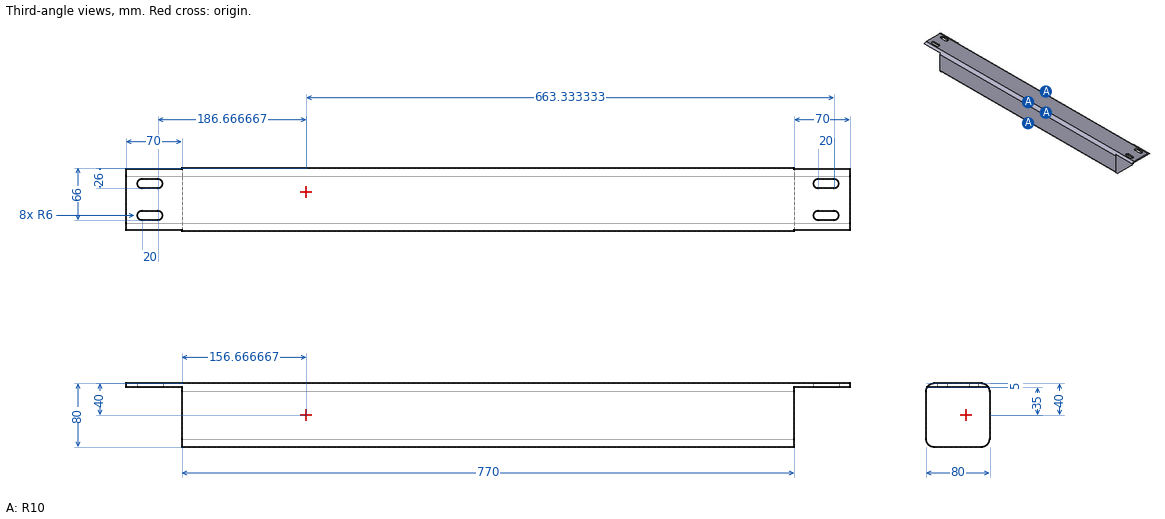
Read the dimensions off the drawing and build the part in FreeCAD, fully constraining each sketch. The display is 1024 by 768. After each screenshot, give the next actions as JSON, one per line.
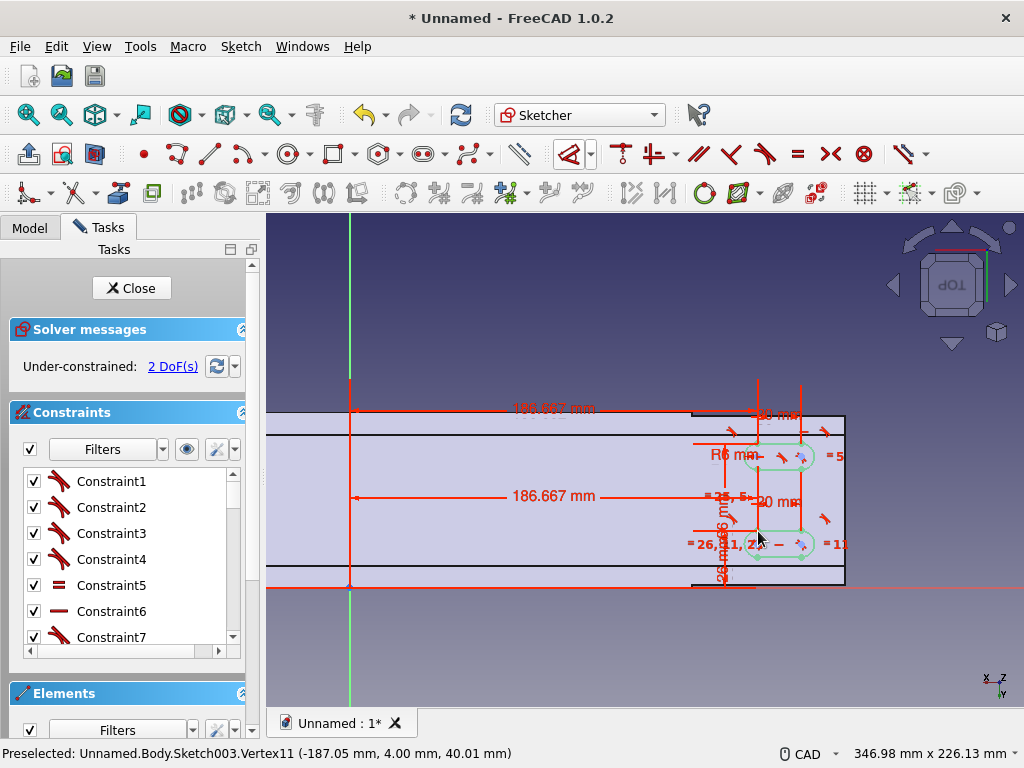
{"action": "scroll", "coordinate": [760, 446], "scroll_direction": "down", "scroll_amount": 8}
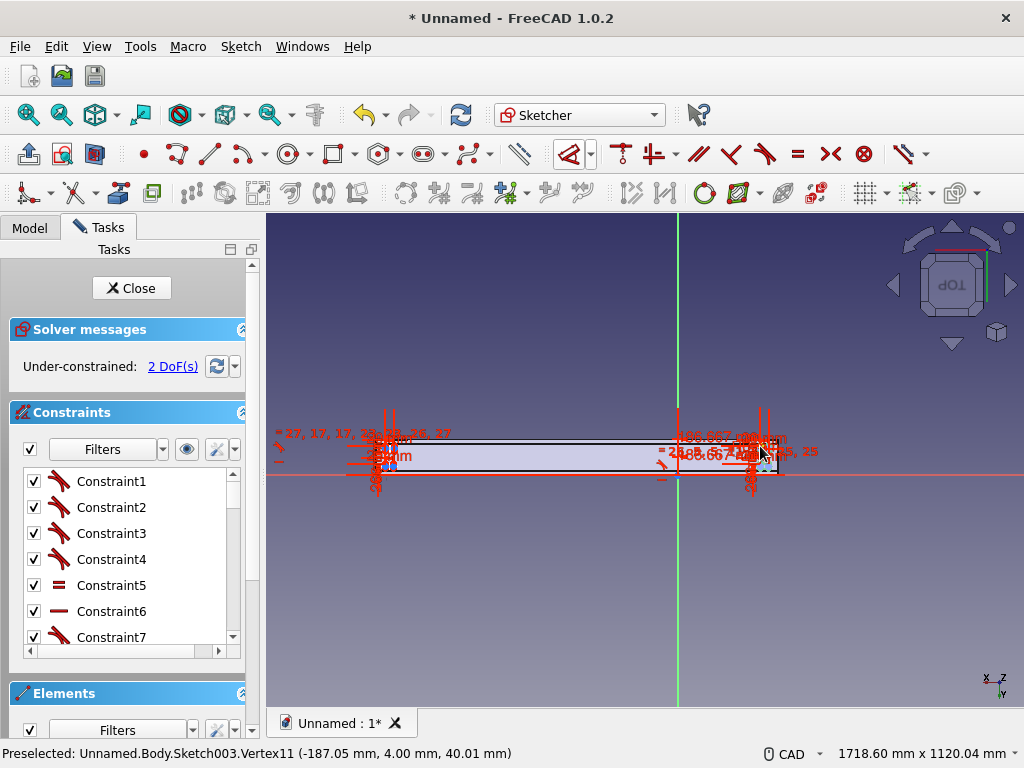
{"action": "scroll", "coordinate": [385, 464], "scroll_direction": "up", "scroll_amount": 8}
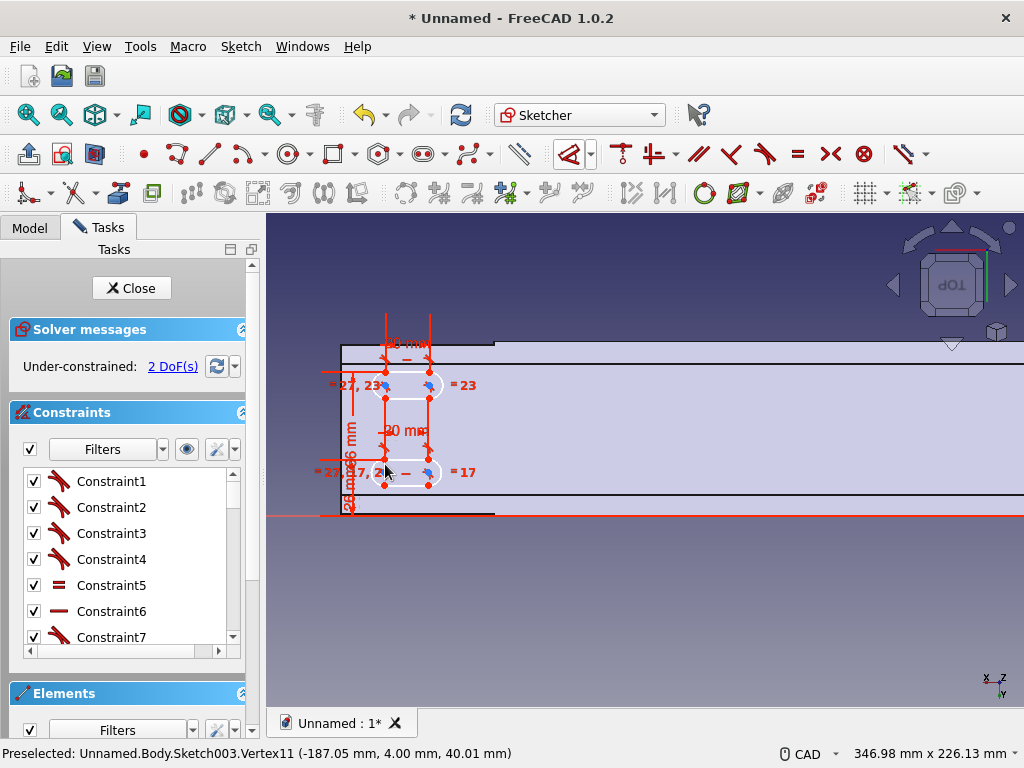
{"action": "left_click", "coordinate": [385, 460]}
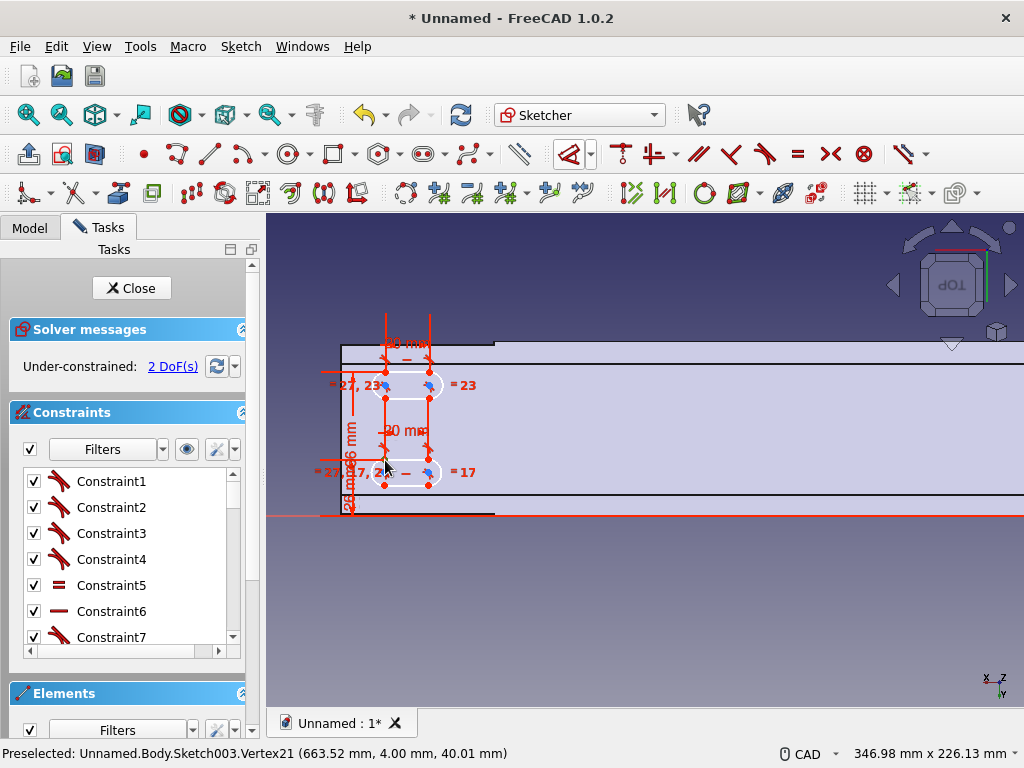
{"action": "left_click", "coordinate": [590, 154]}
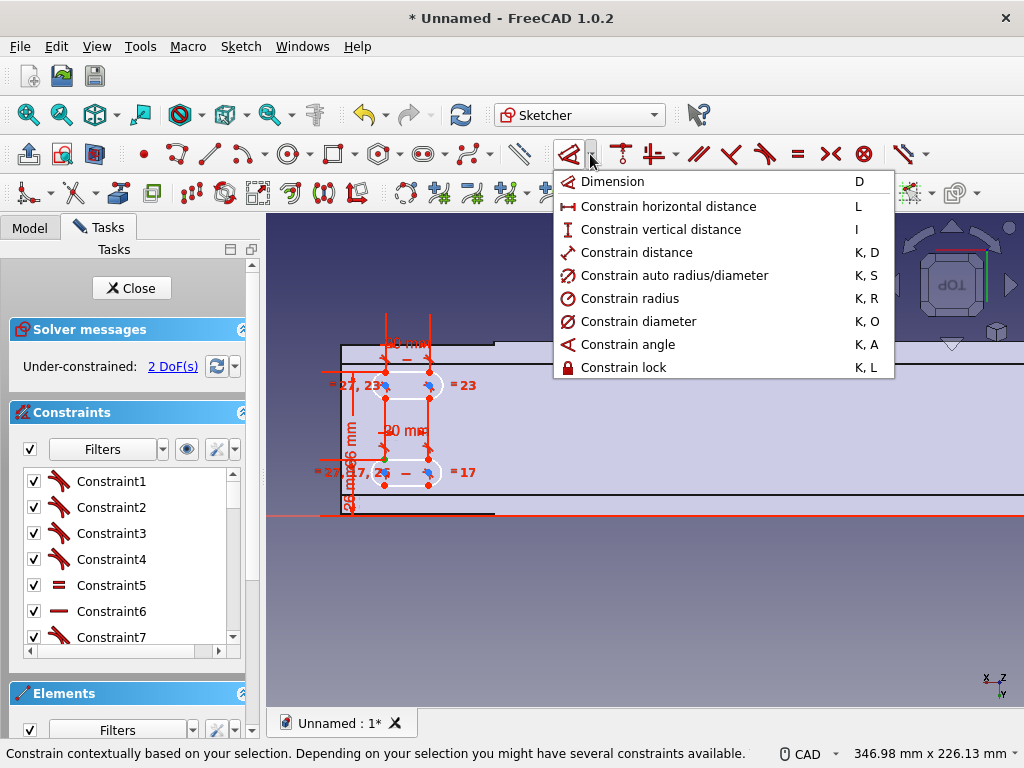
{"action": "left_click", "coordinate": [724, 206]}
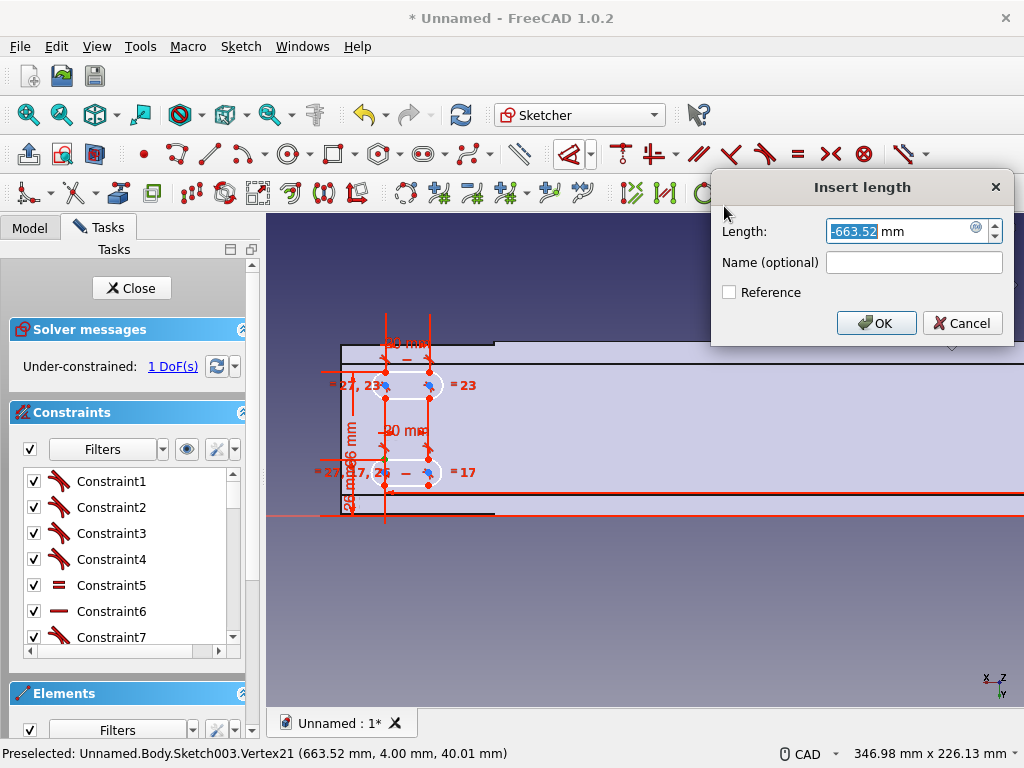
{"action": "type", "text": "-663.333333"}
{"action": "key", "text": "Return"}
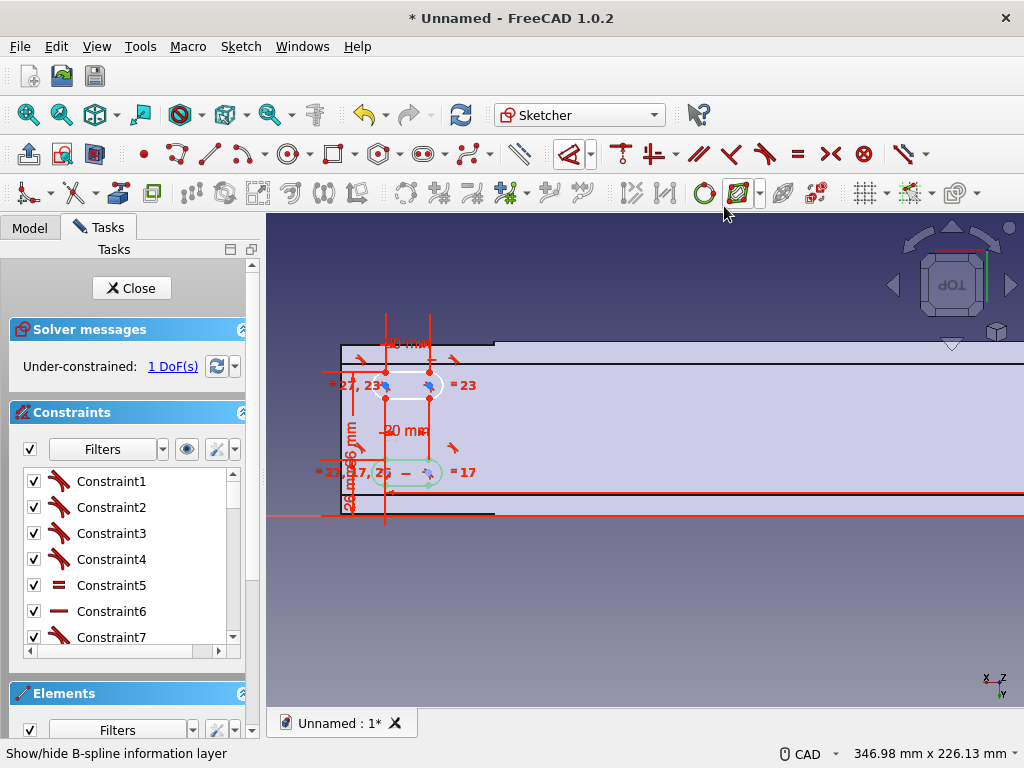
{"action": "left_click", "coordinate": [386, 372]}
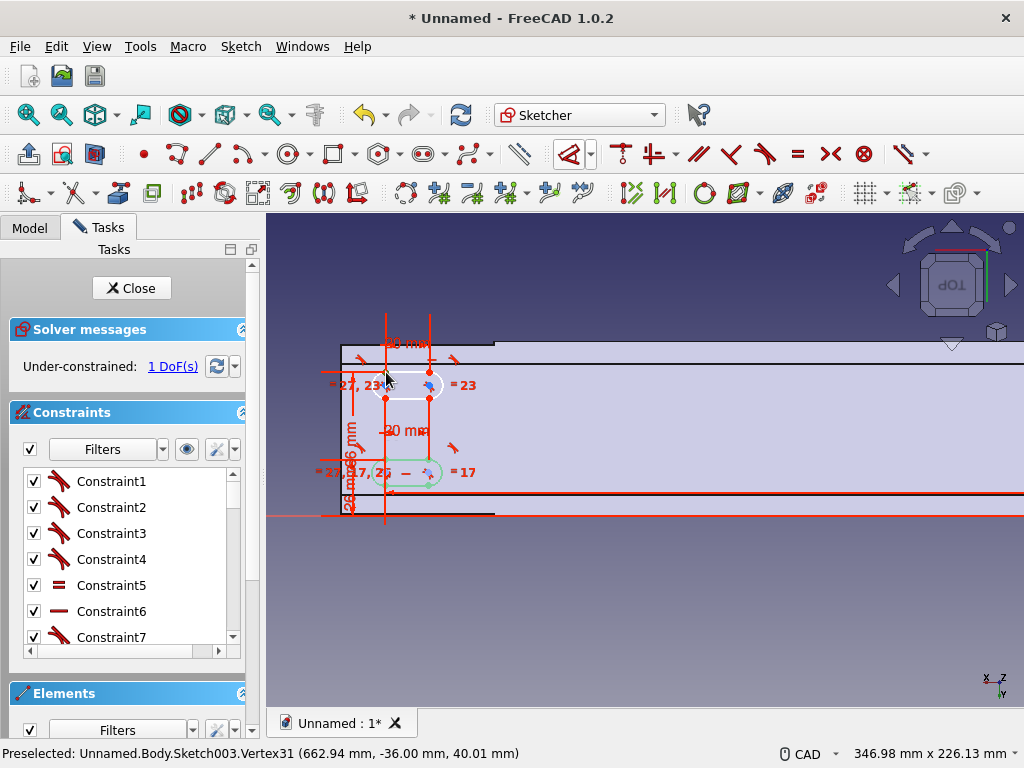
{"action": "left_click", "coordinate": [590, 154]}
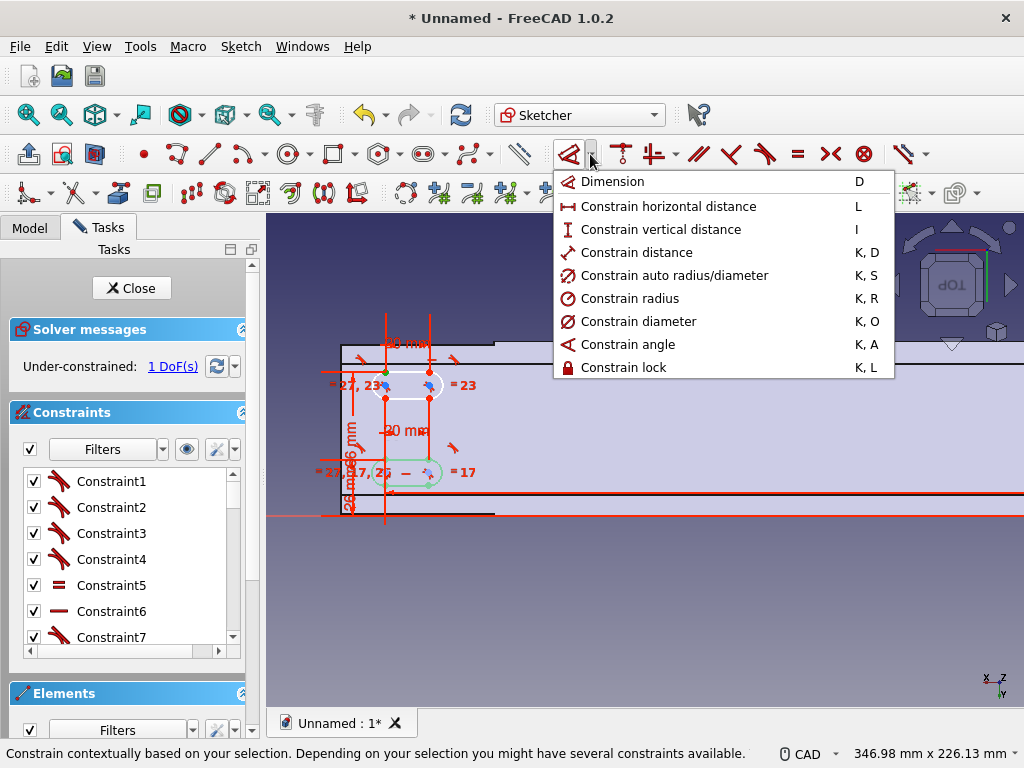
{"action": "left_click", "coordinate": [724, 206]}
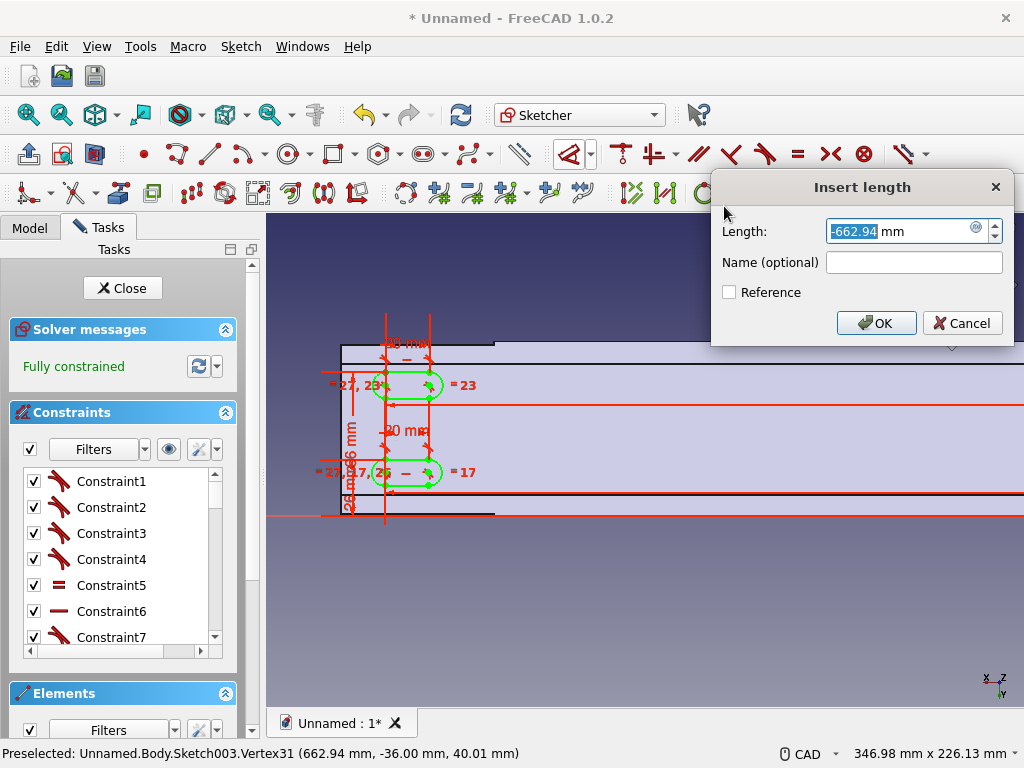
{"action": "type", "text": "-663.333333"}
{"action": "key", "text": "Return"}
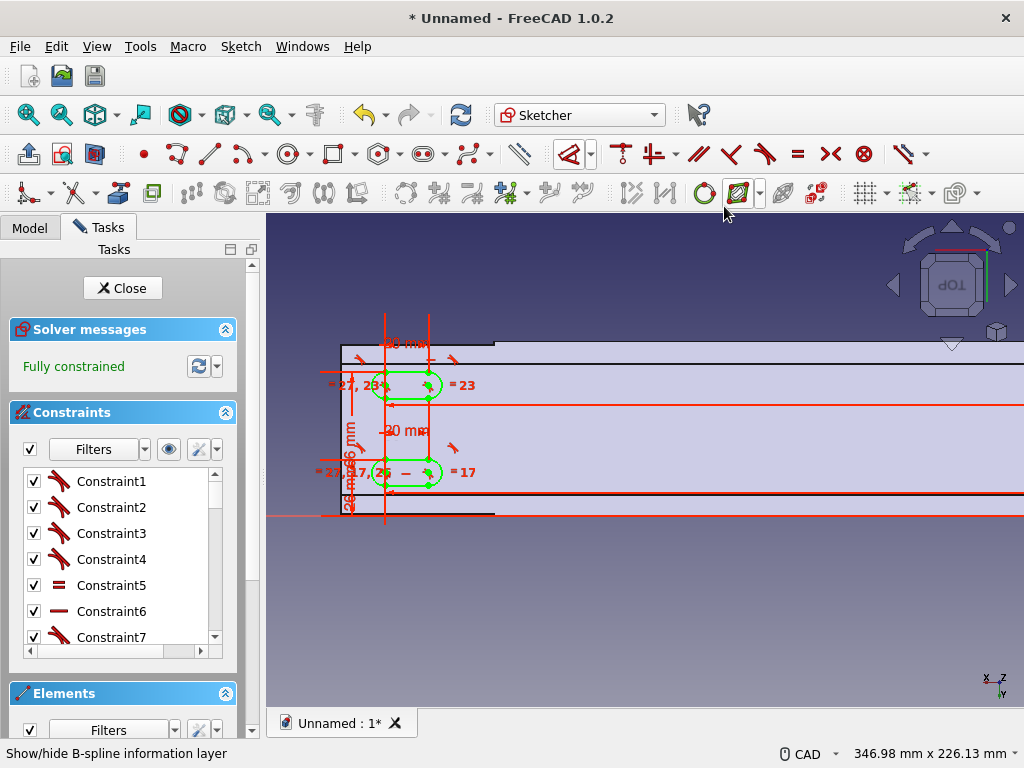
{"action": "left_click", "coordinate": [123, 288]}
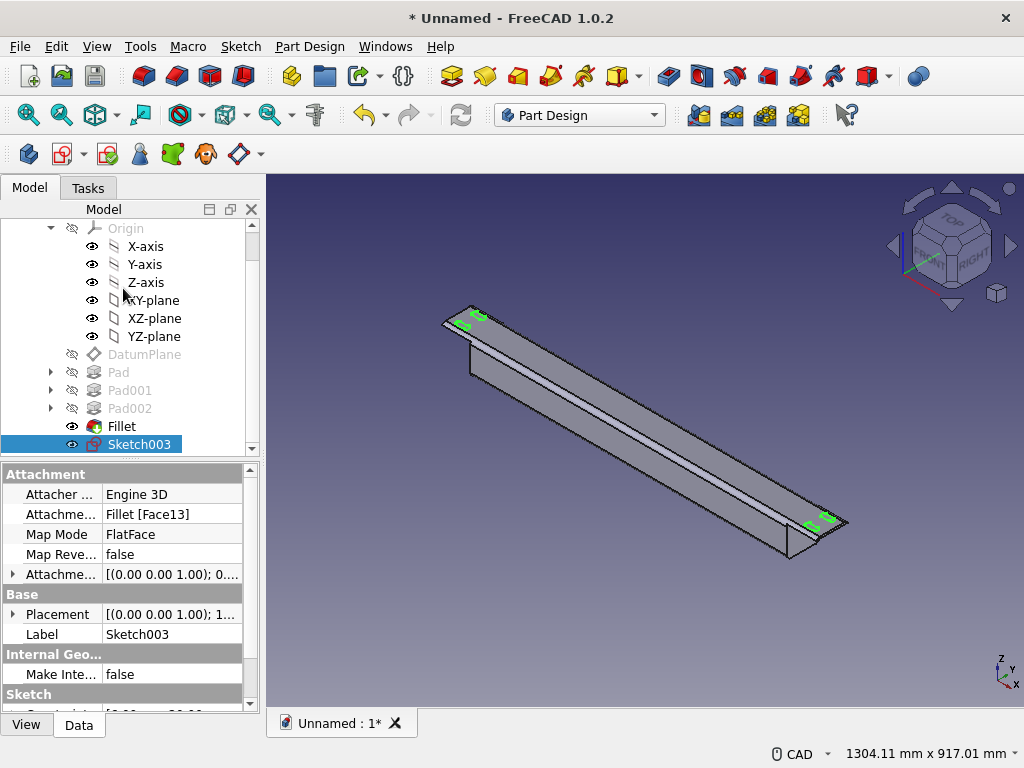
{"action": "left_click", "coordinate": [669, 76]}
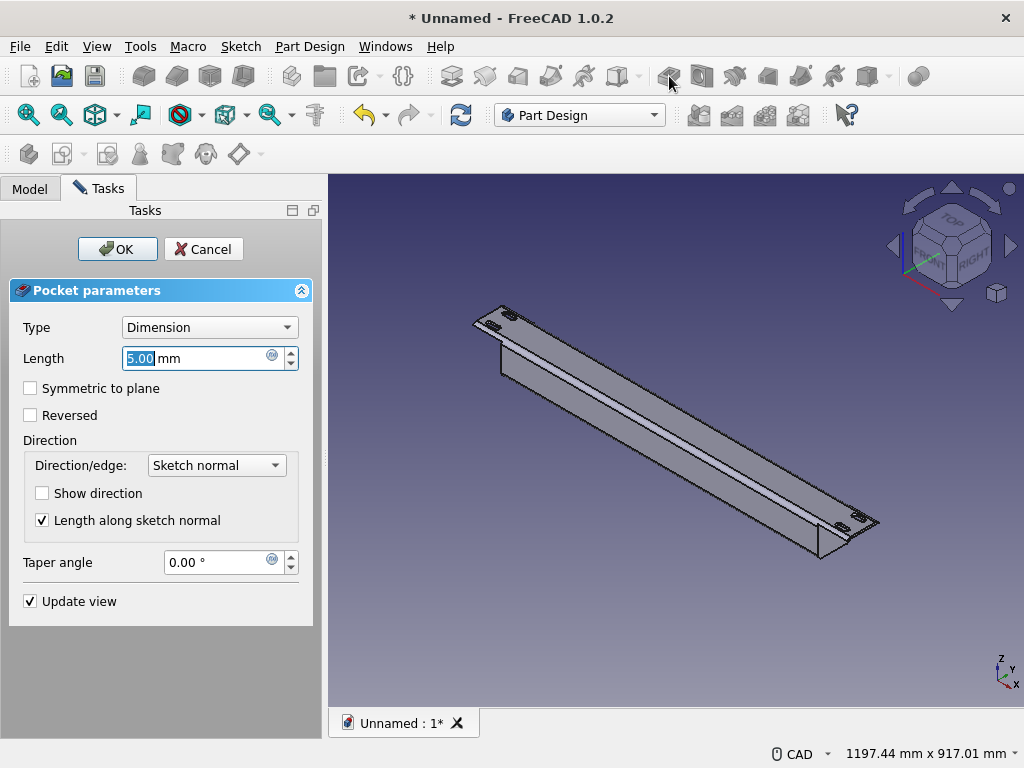
{"action": "left_click", "coordinate": [210, 328]}